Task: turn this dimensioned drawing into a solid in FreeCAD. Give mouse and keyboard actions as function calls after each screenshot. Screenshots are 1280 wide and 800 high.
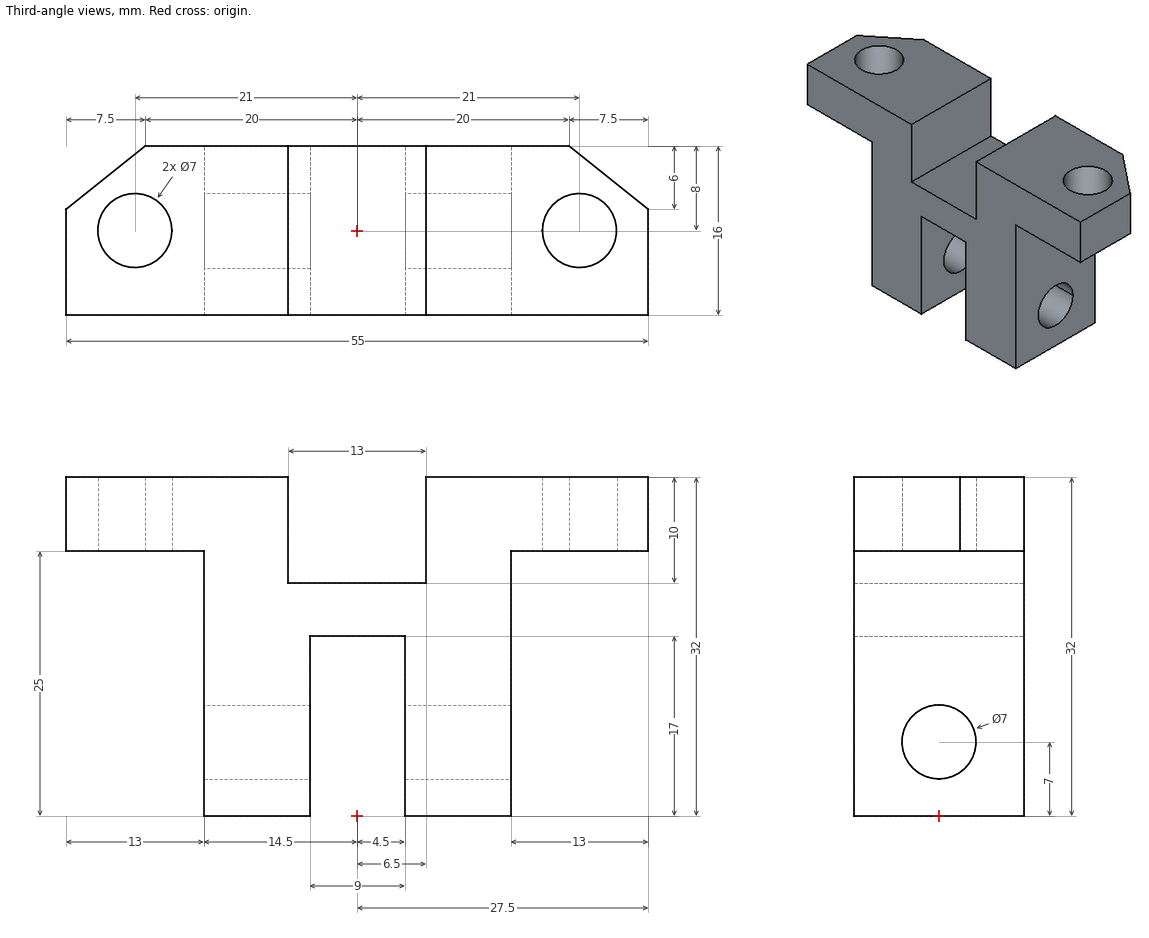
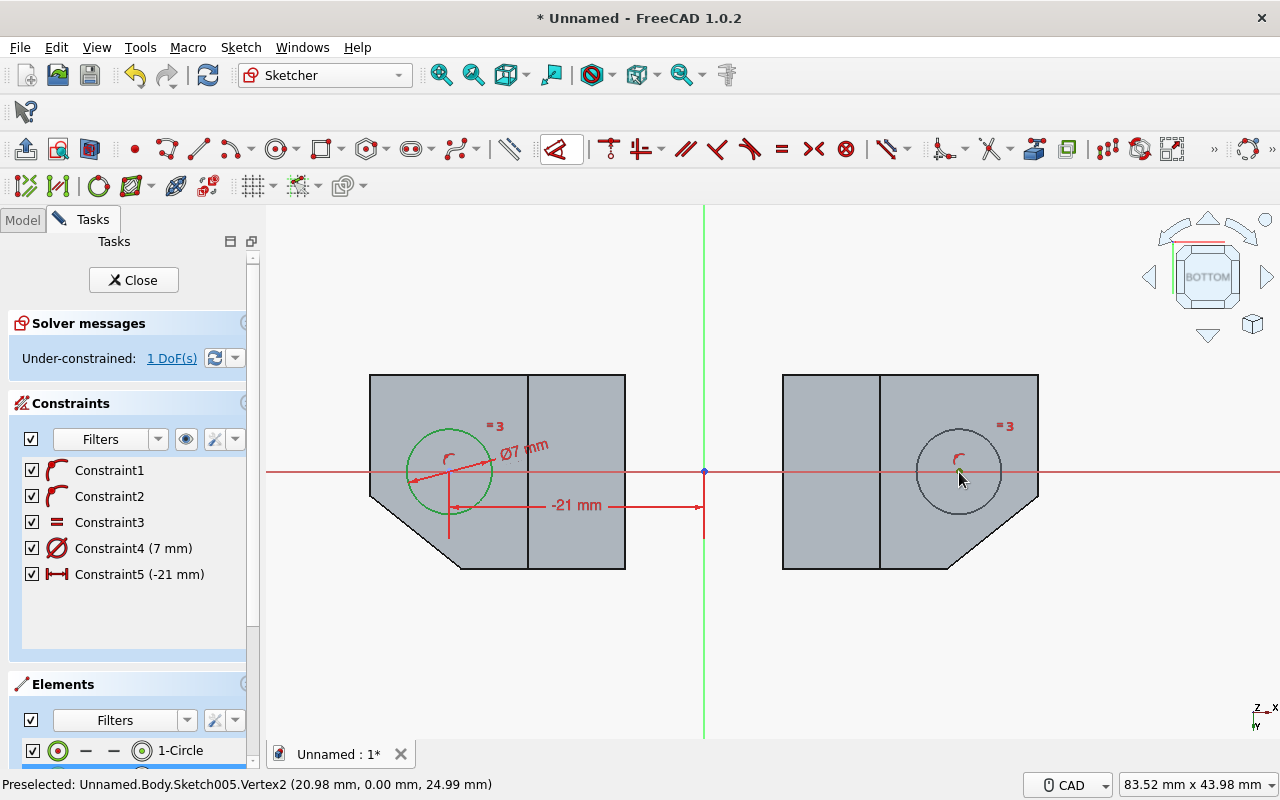
click(578, 150)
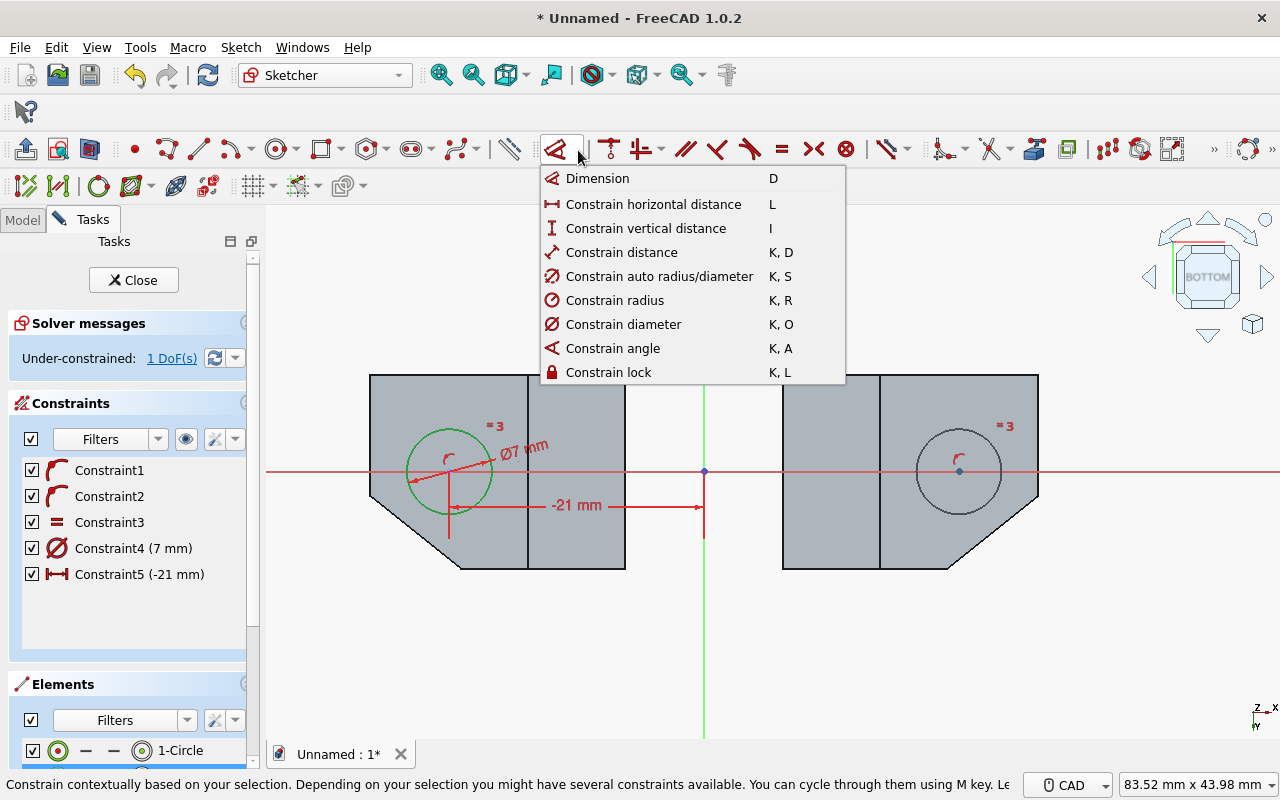
click(693, 204)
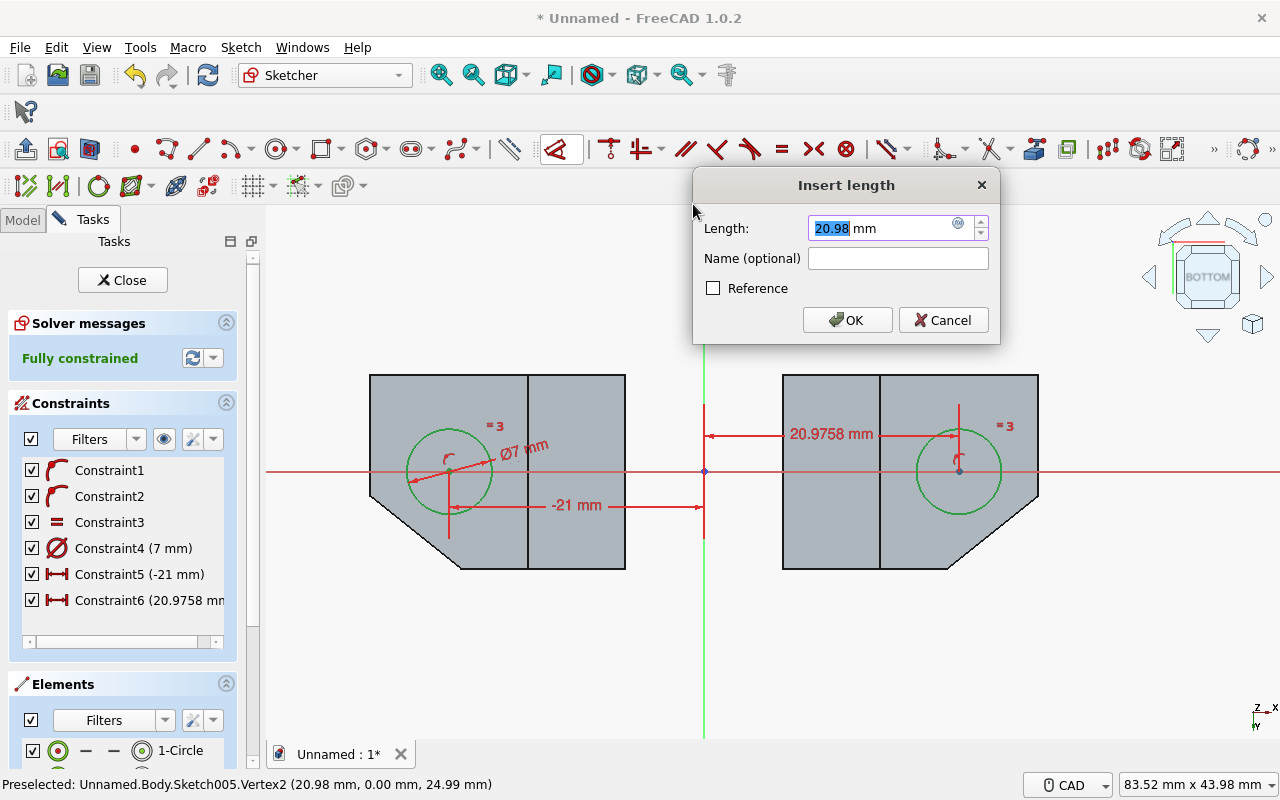
text(21)
key(Return)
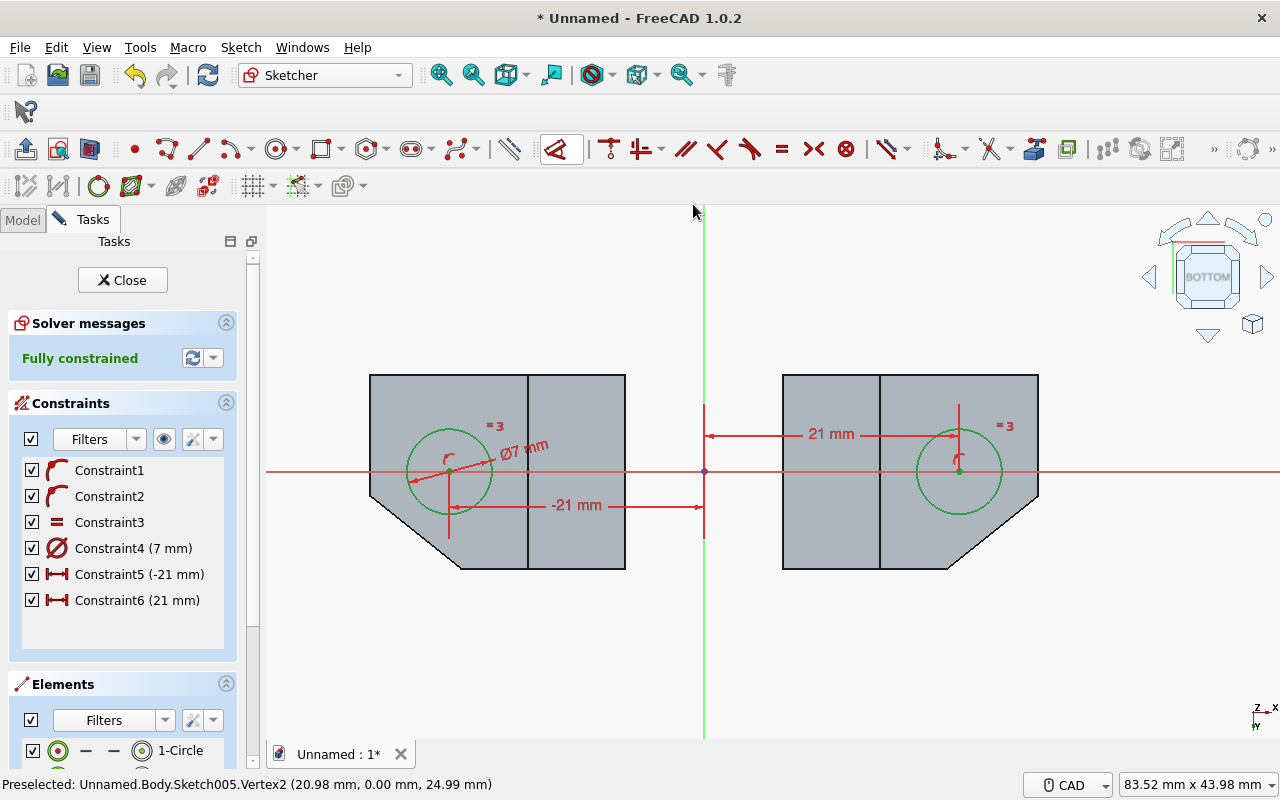
click(123, 280)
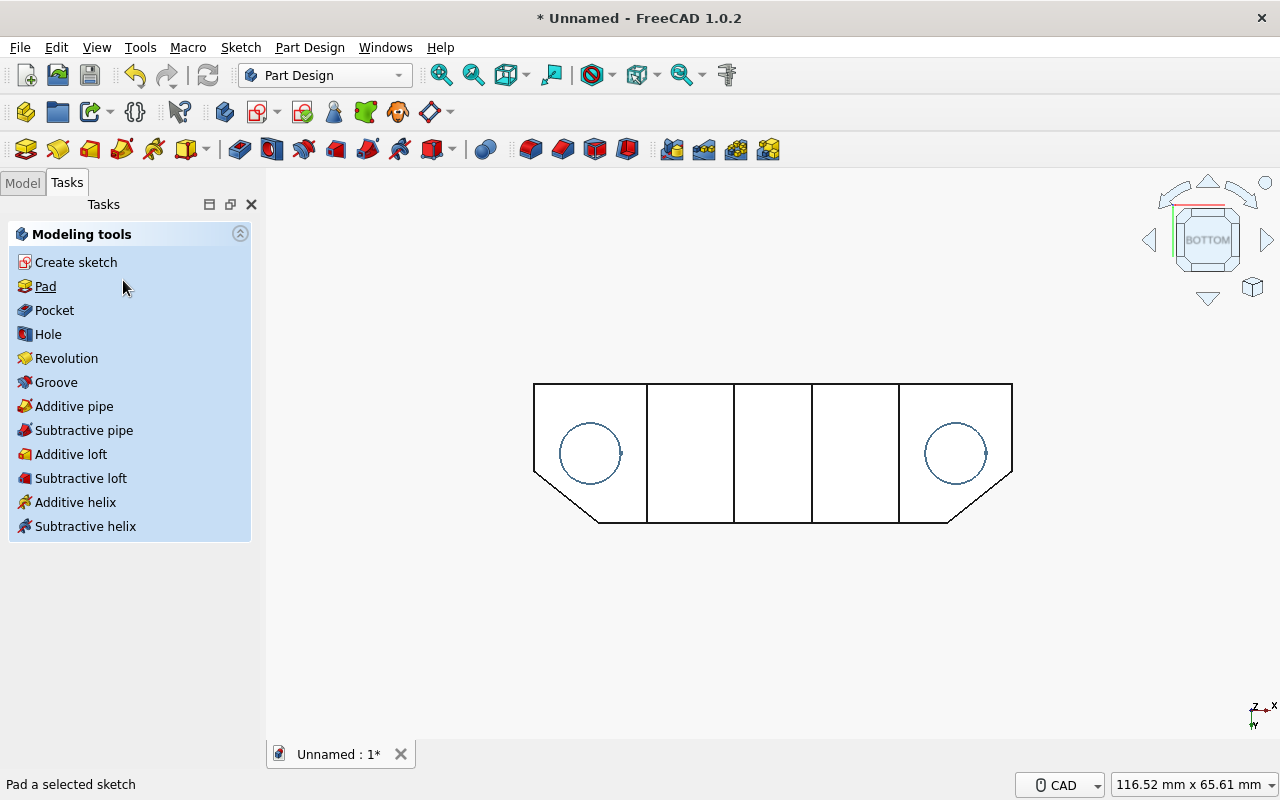
click(240, 150)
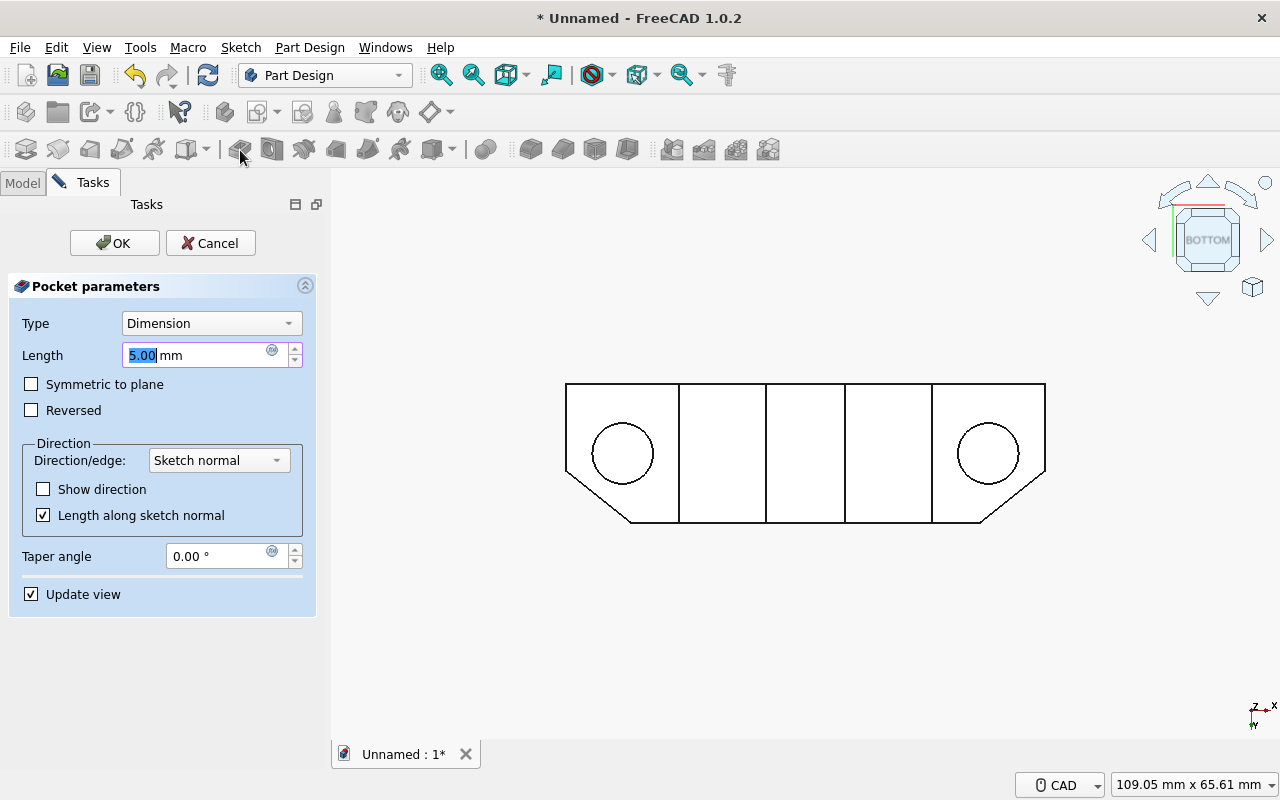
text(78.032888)
key(Tab)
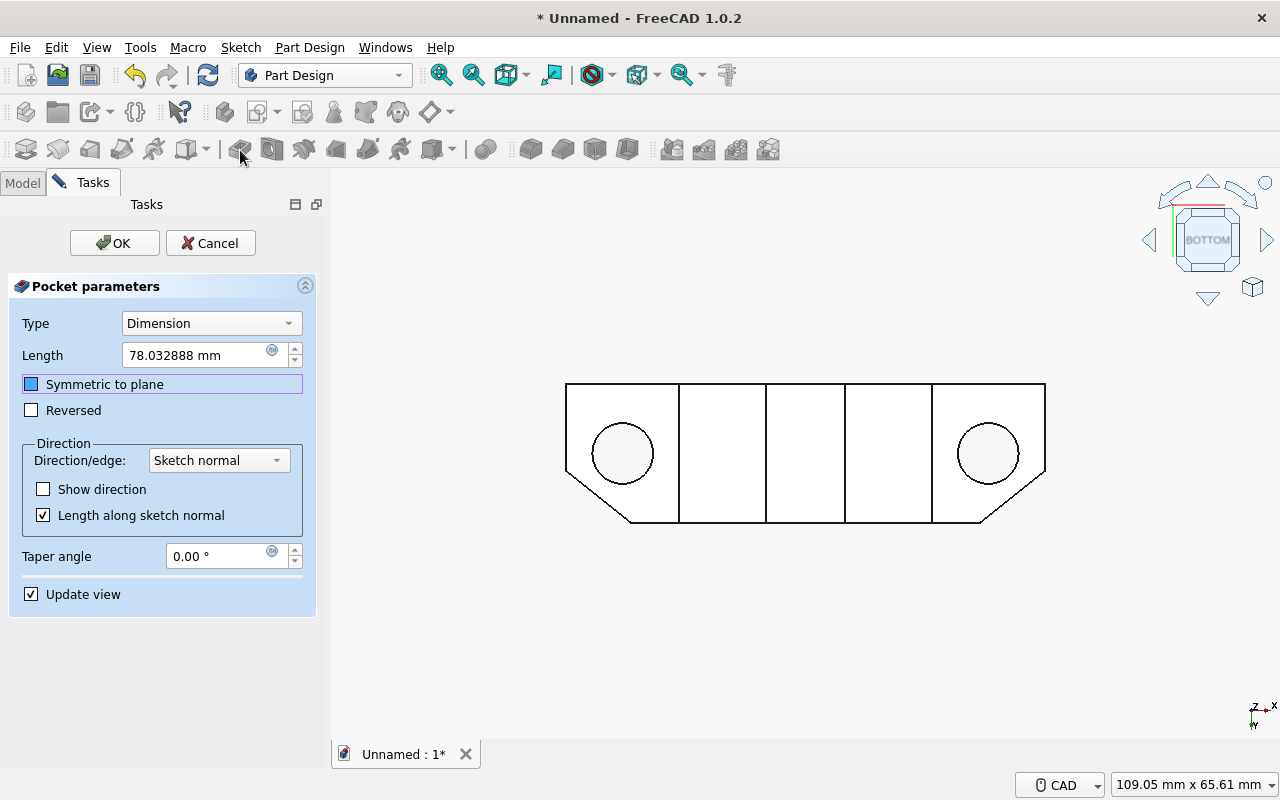
click(30, 384)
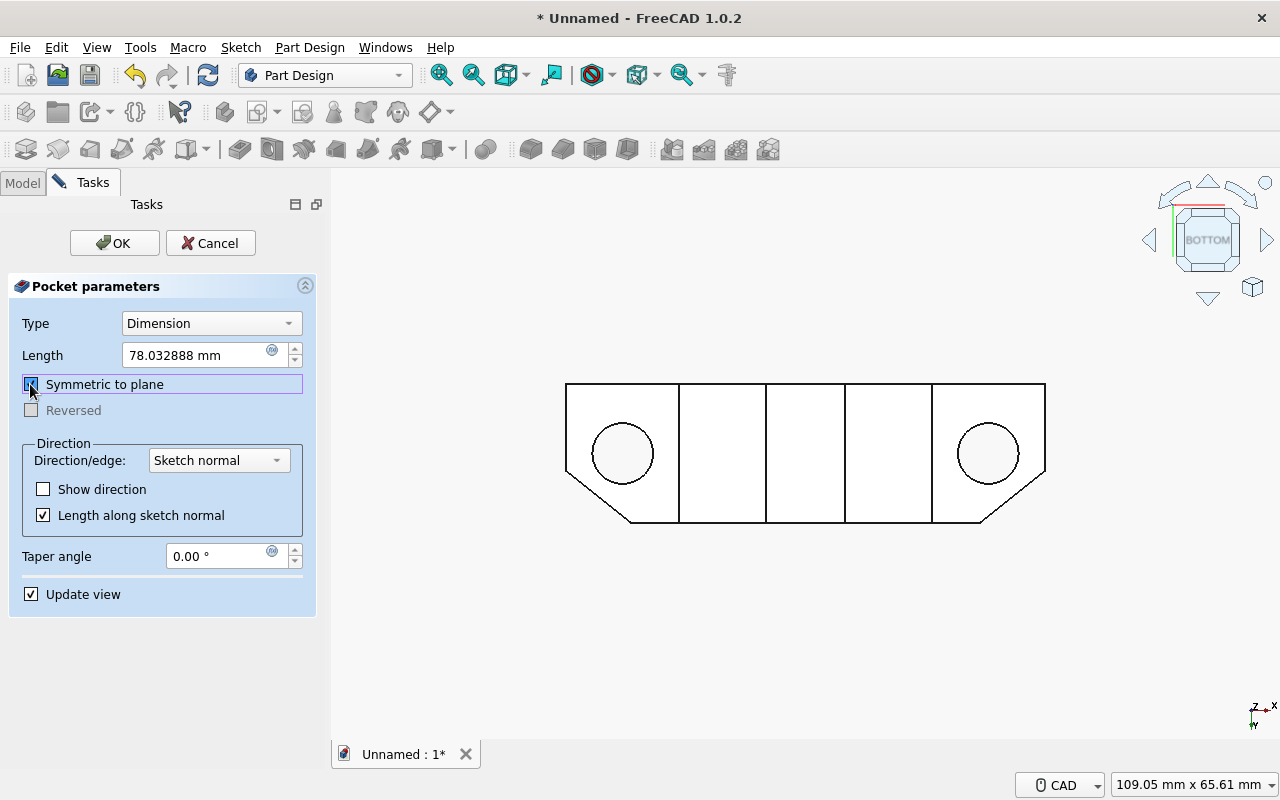
click(115, 243)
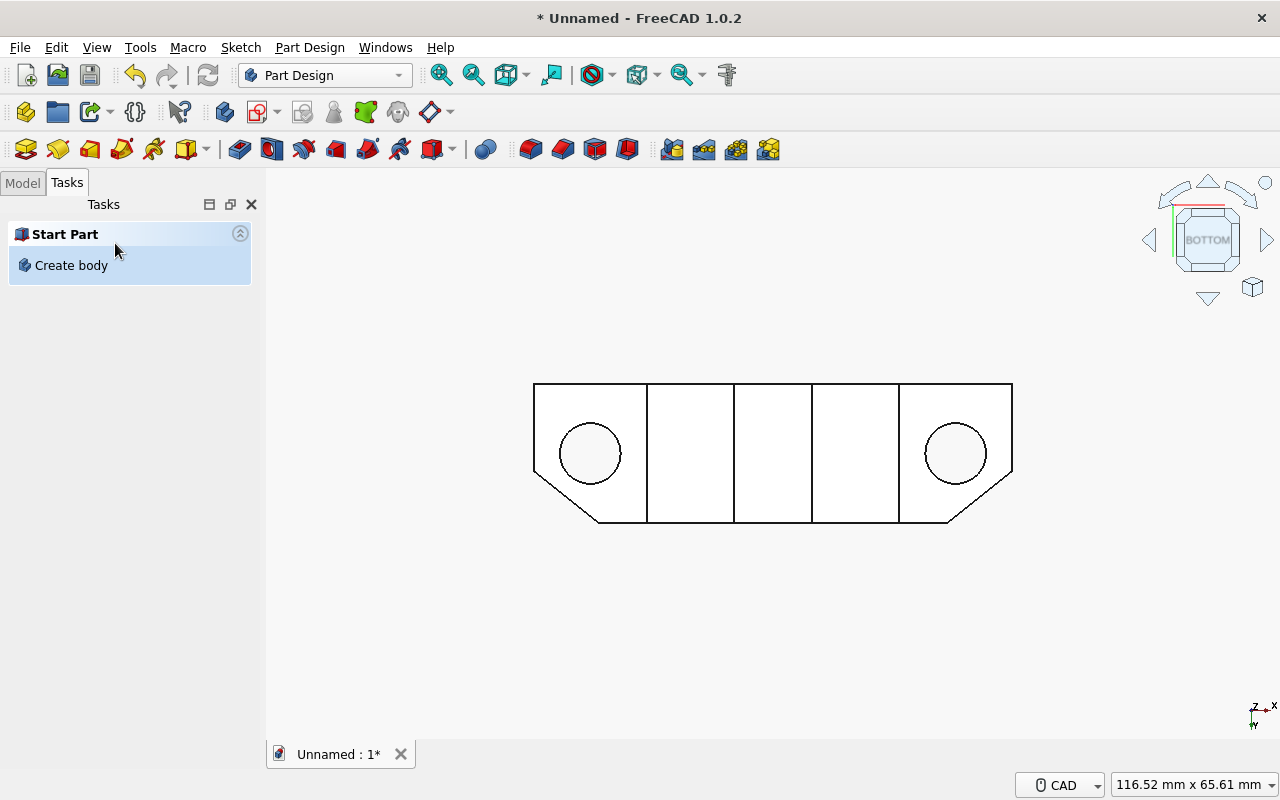
key(0)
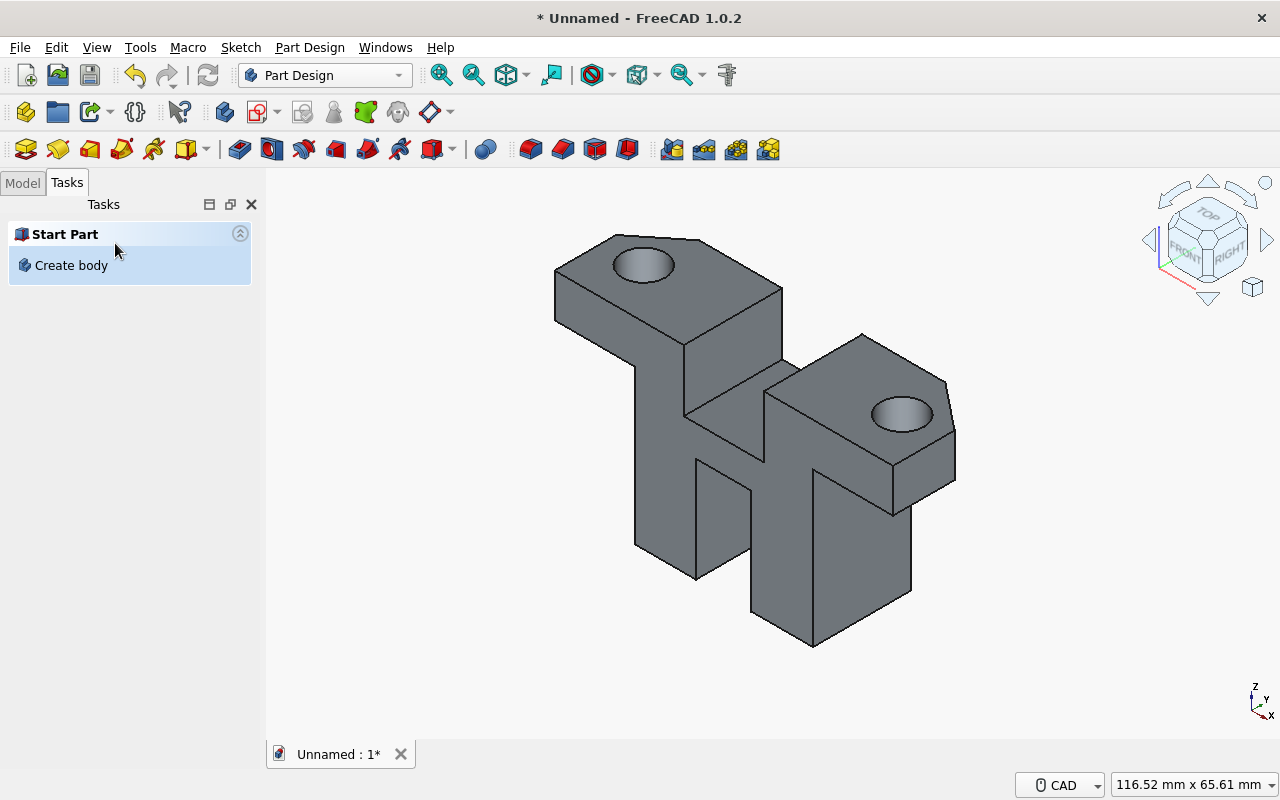
click(862, 529)